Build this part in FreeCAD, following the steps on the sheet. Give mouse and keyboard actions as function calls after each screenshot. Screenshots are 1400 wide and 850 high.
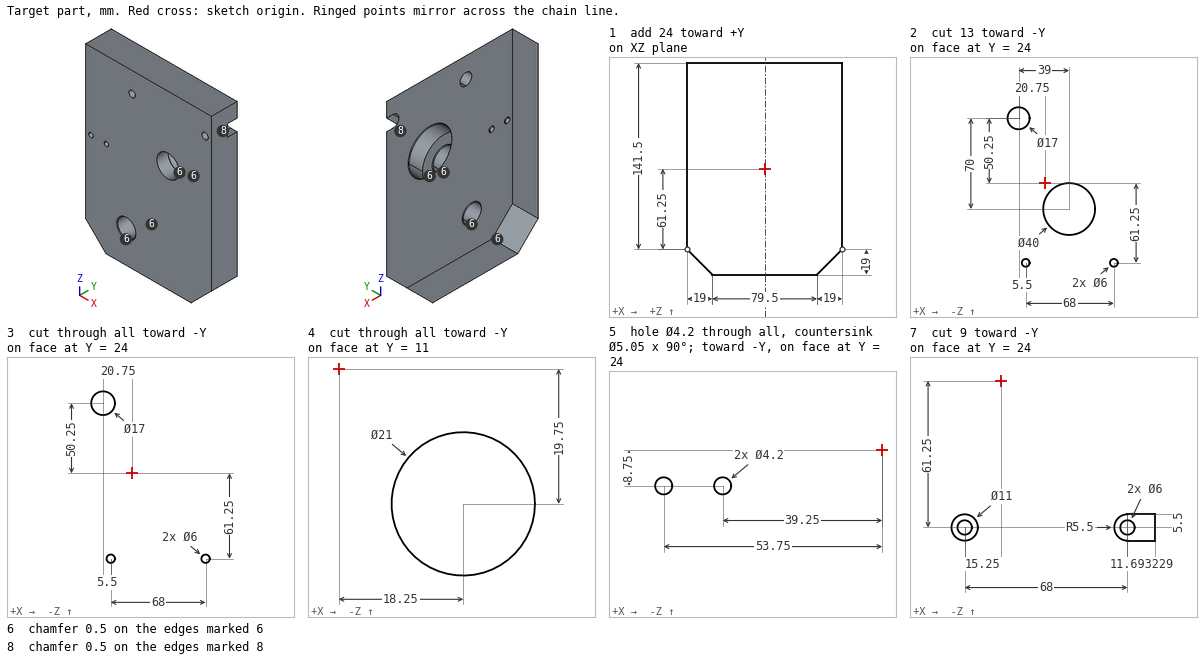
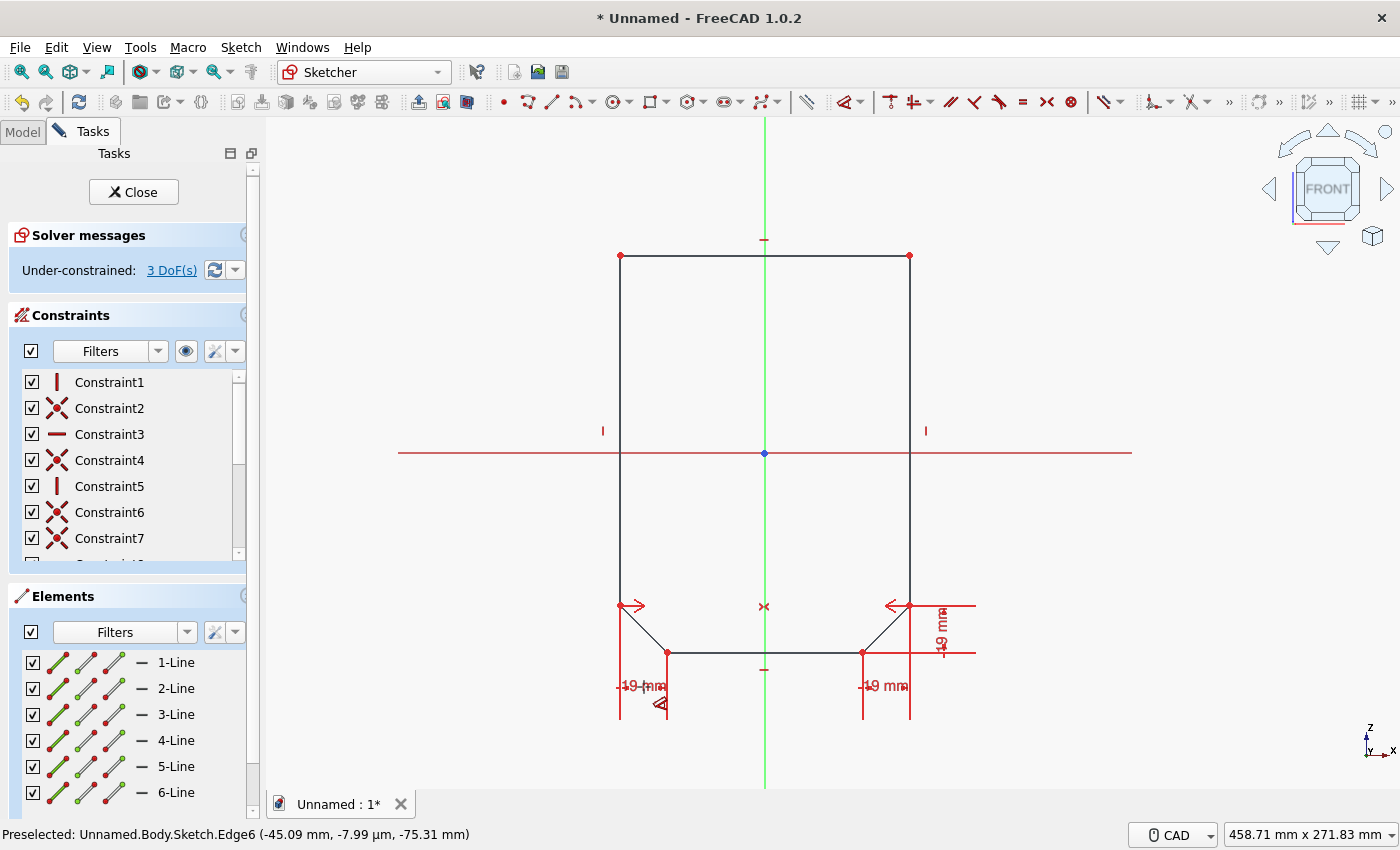
click(804, 653)
click(720, 687)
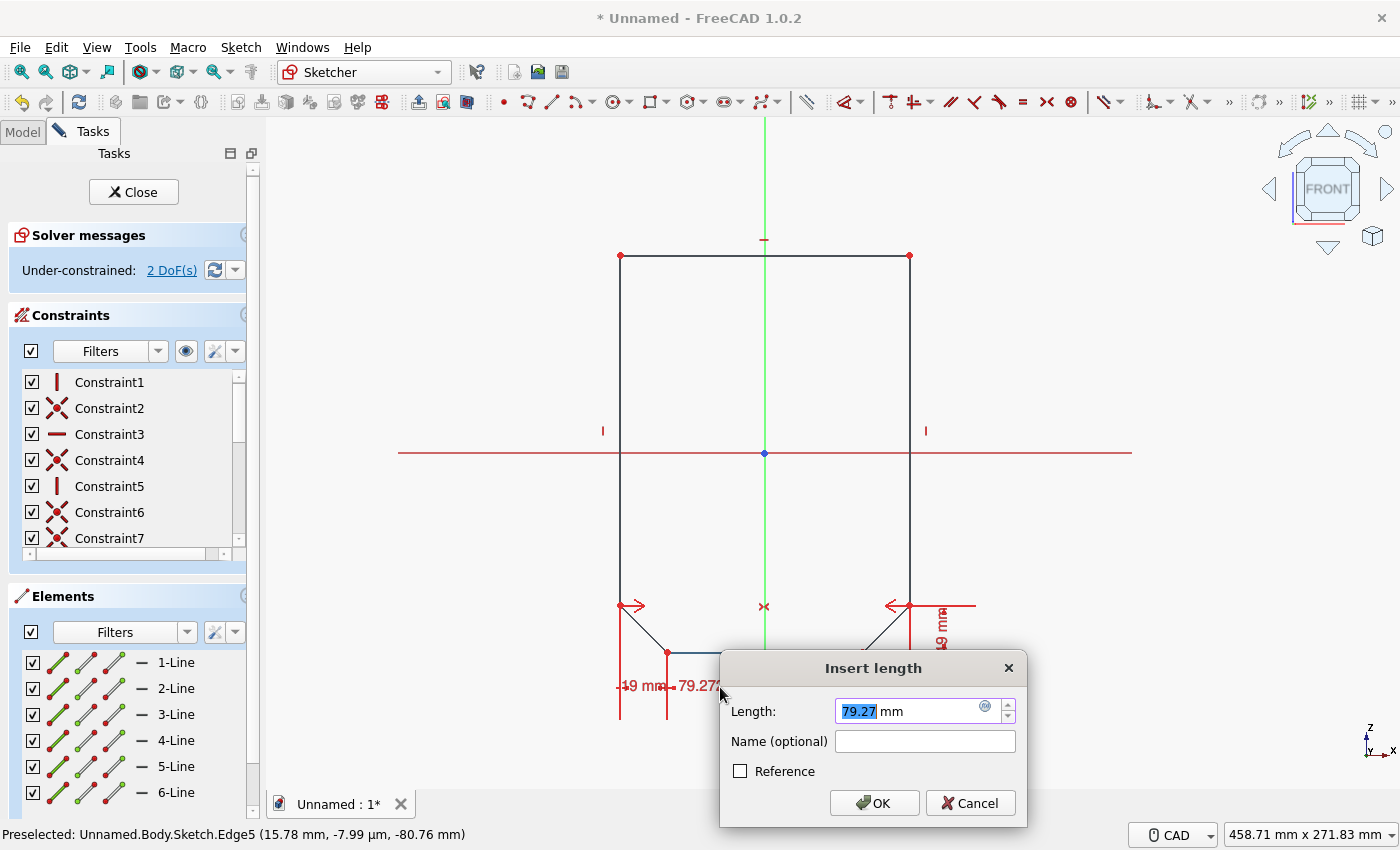
text(79.5)
key(Return)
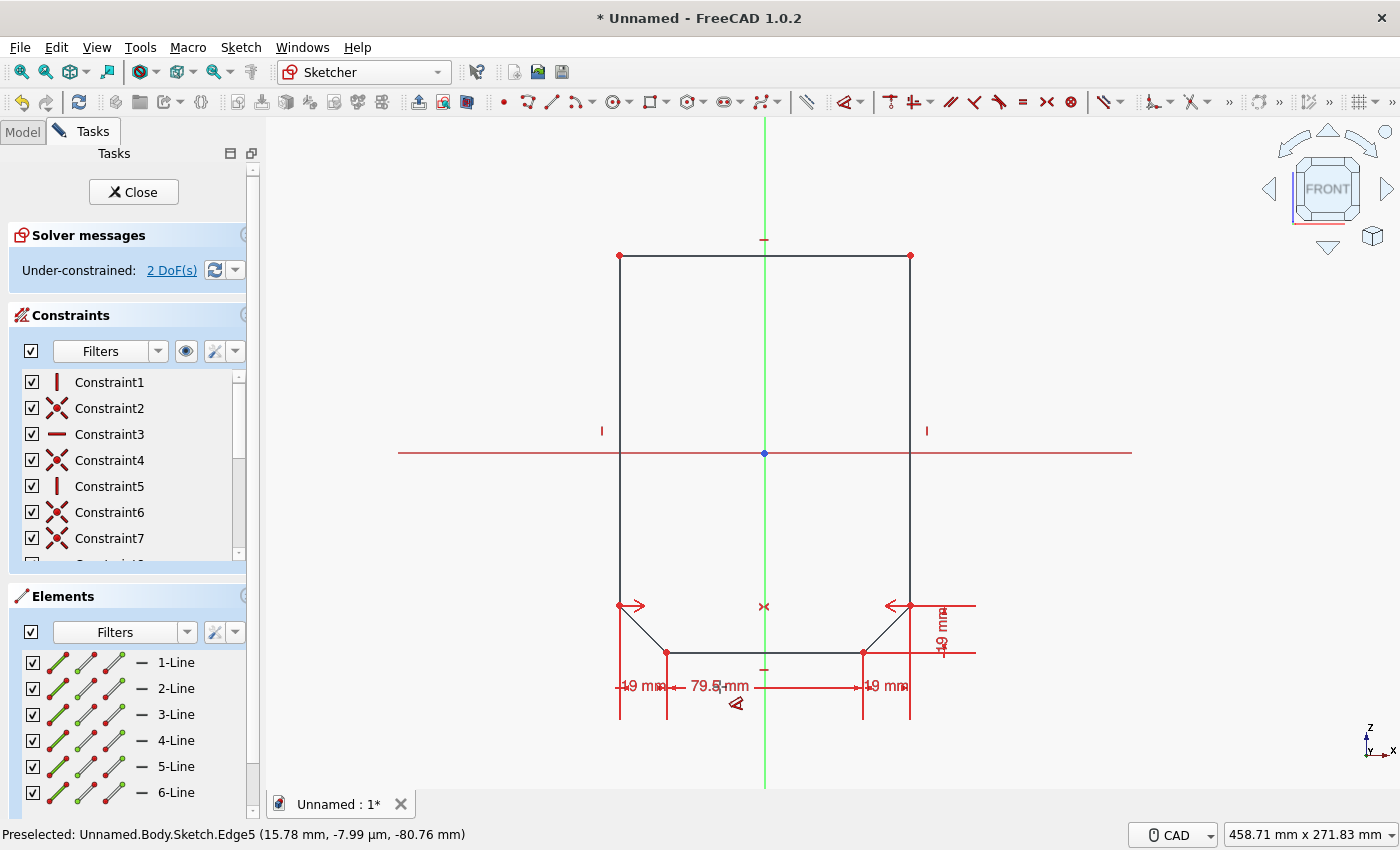
click(620, 501)
click(586, 431)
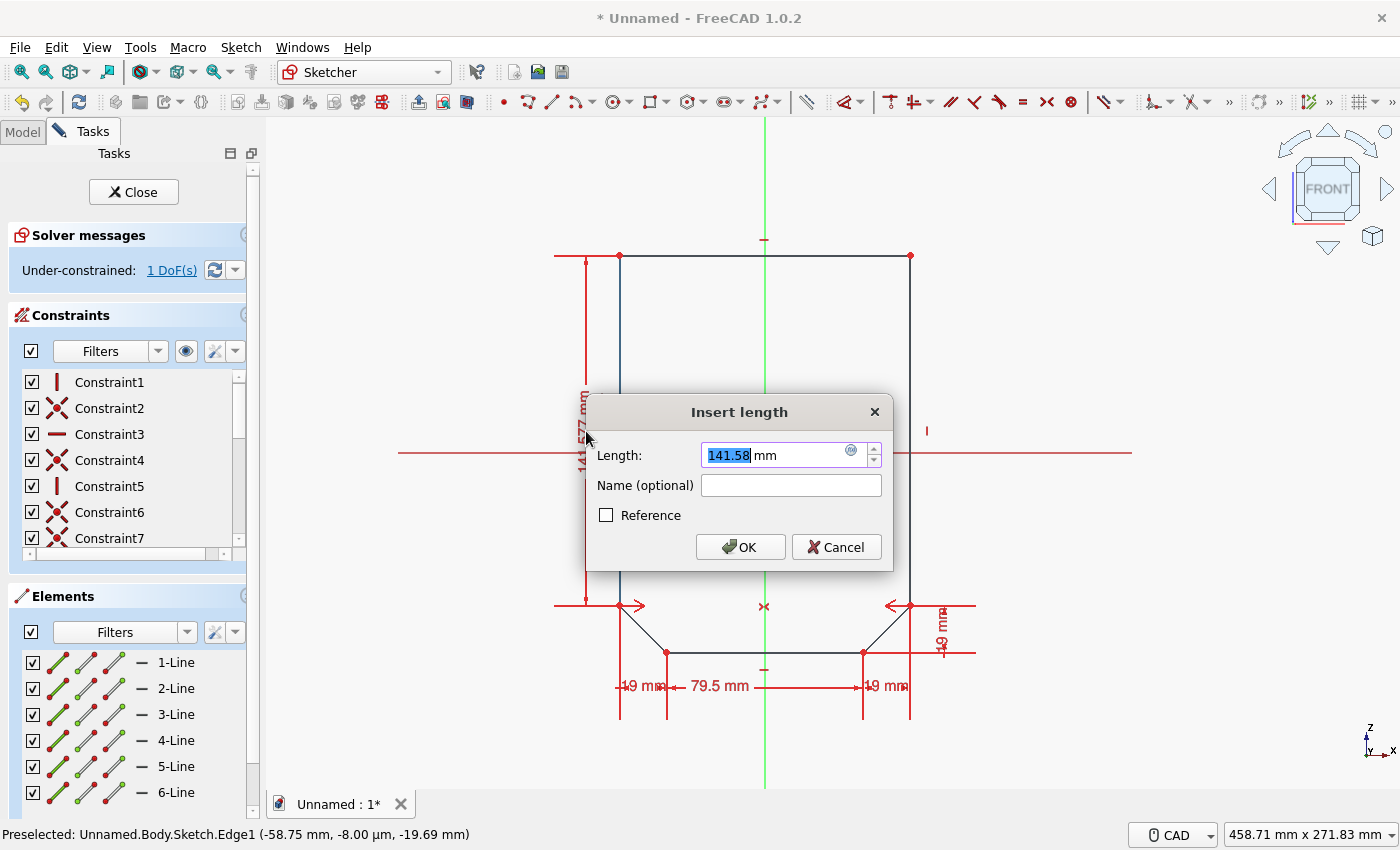
text(141.5)
key(Return)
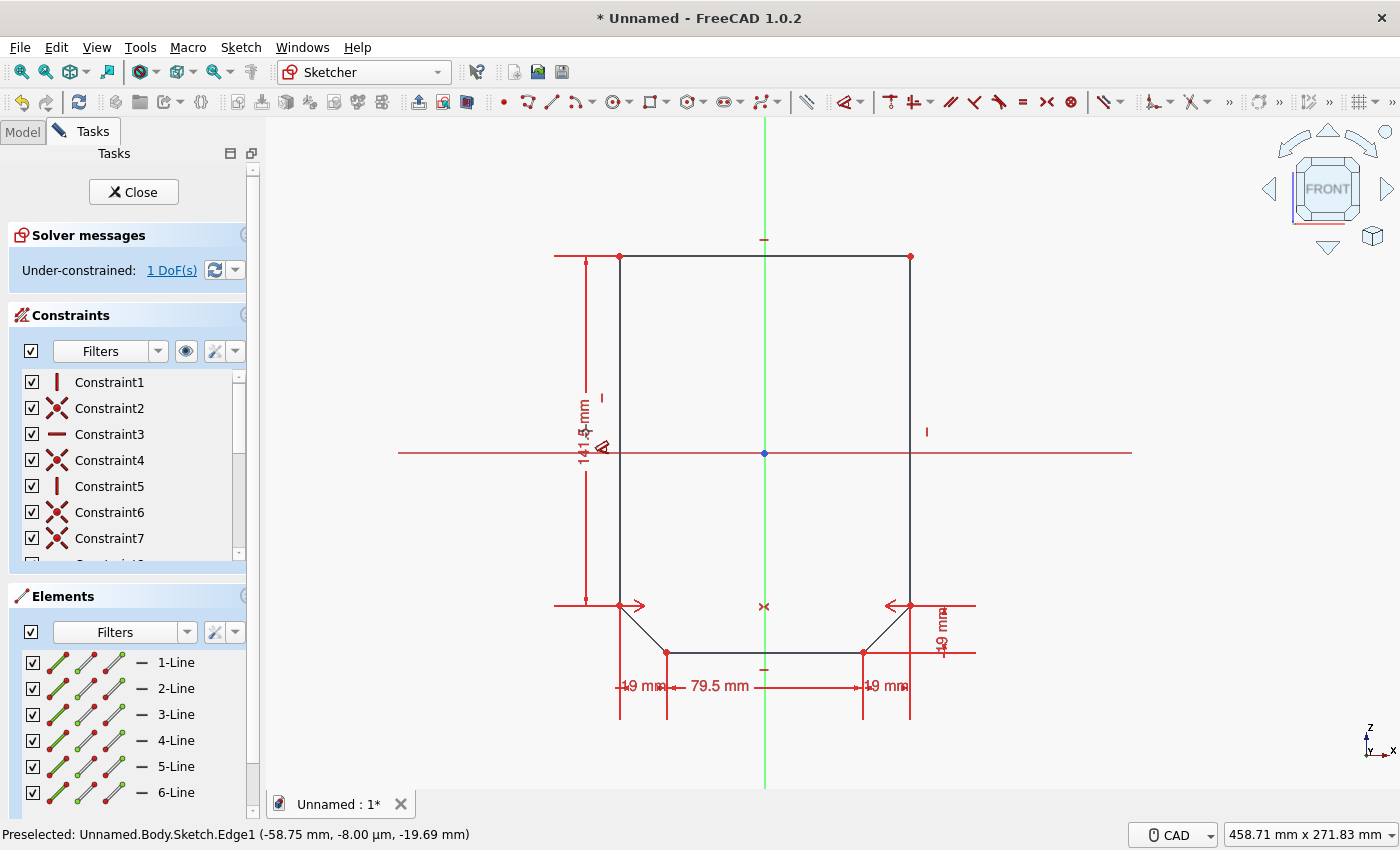
click(620, 606)
click(586, 530)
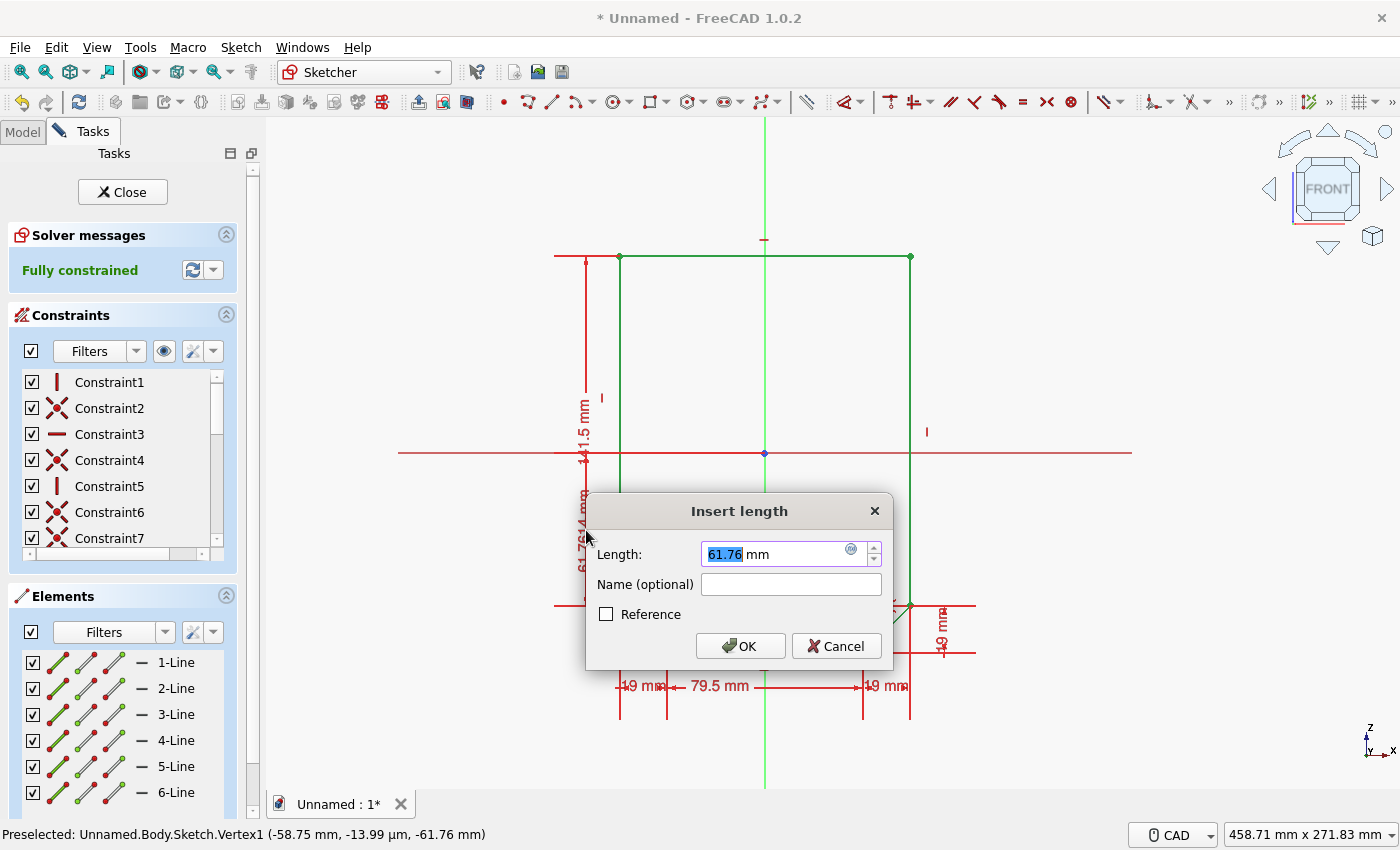
text(61.25)
key(Return)
key(Escape)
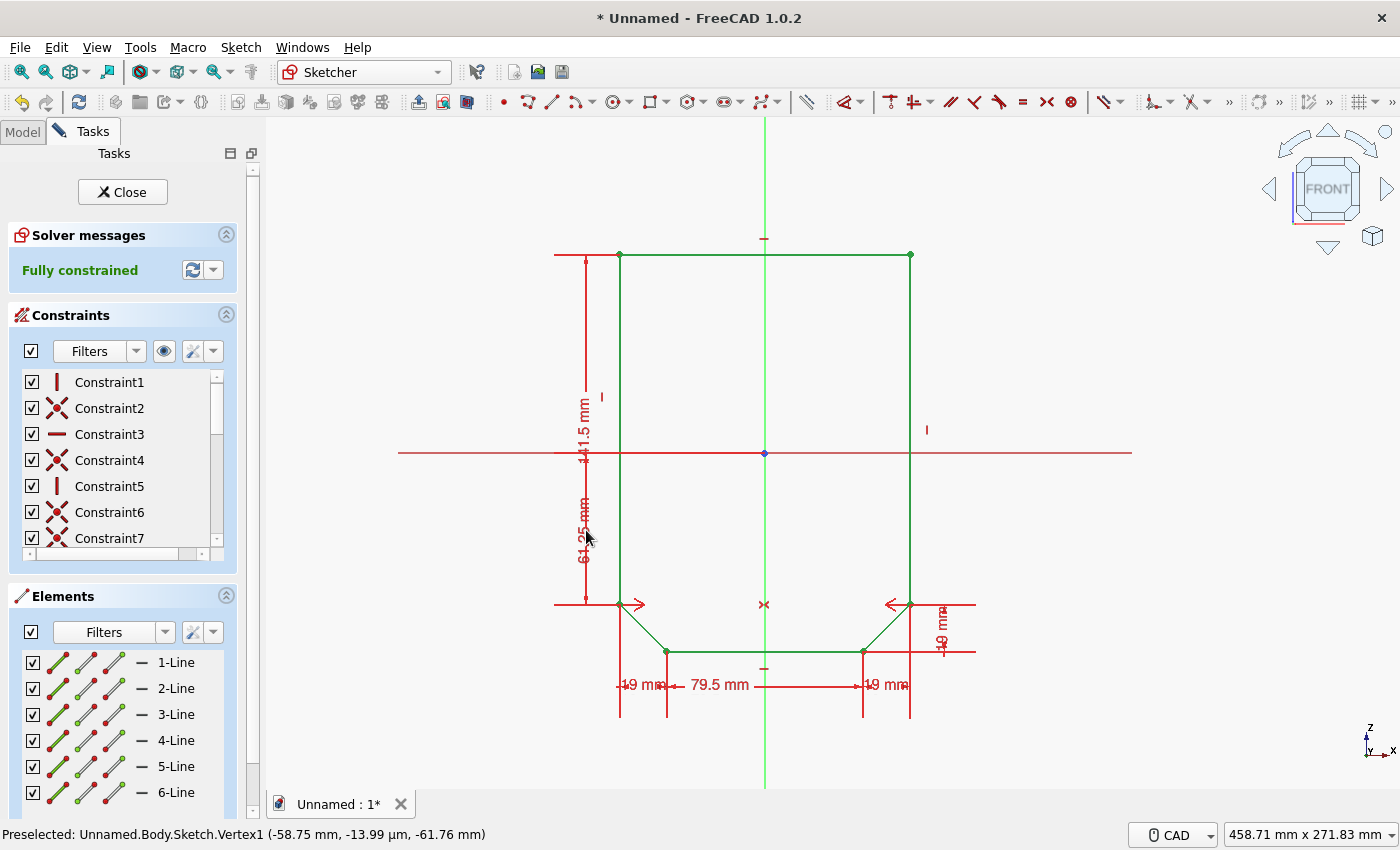
click(123, 192)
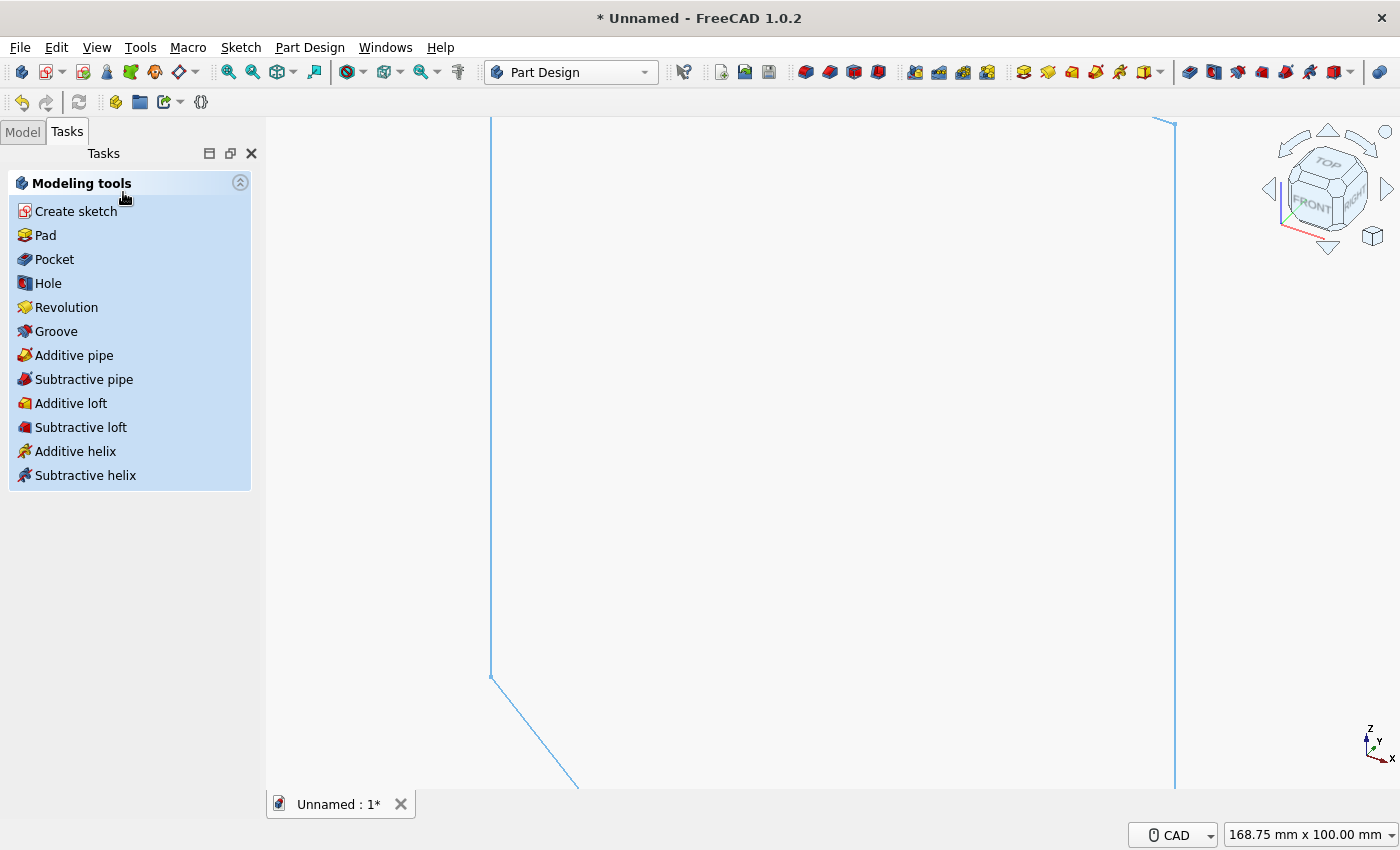
click(1024, 72)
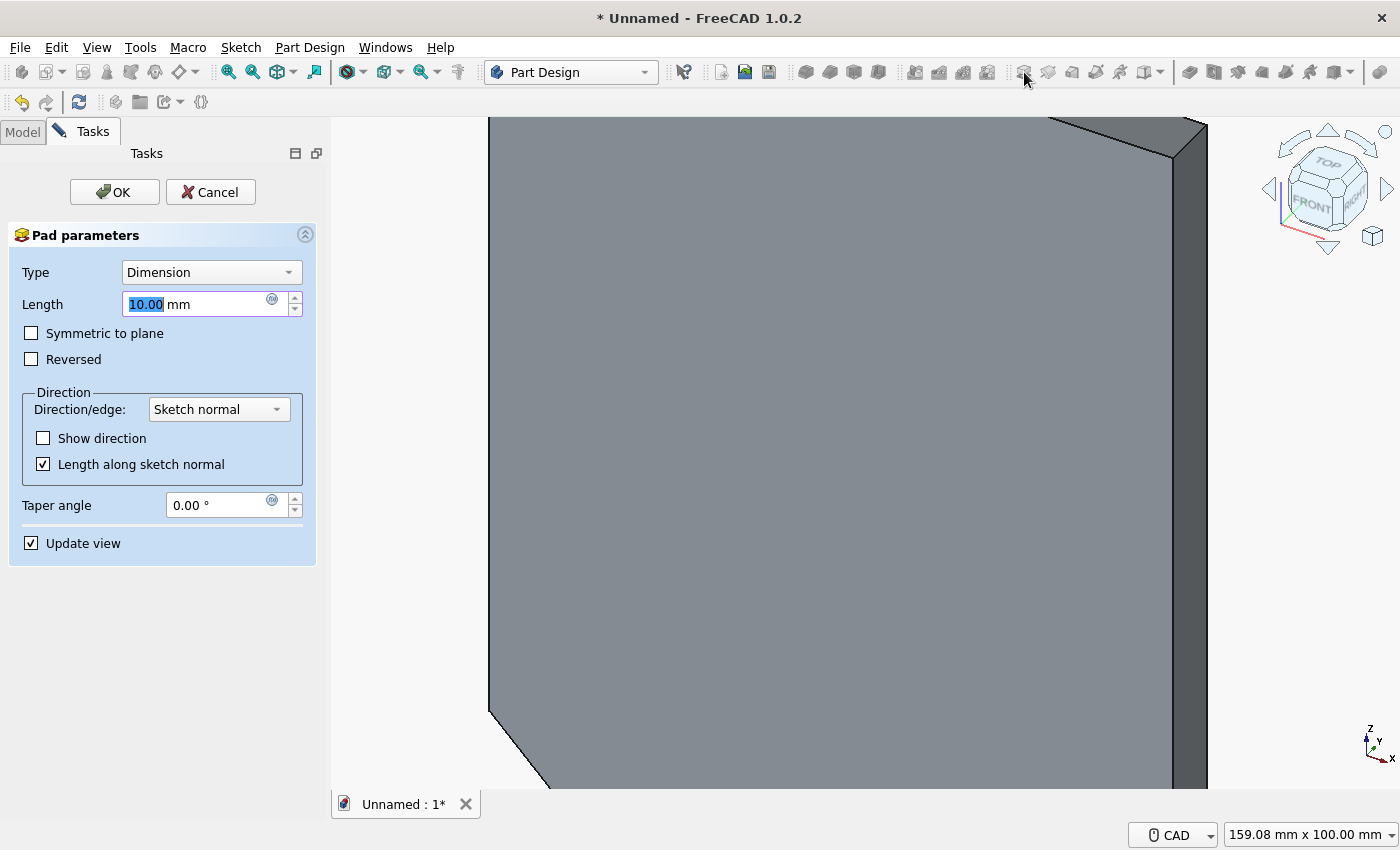
text(24)
key(Tab)